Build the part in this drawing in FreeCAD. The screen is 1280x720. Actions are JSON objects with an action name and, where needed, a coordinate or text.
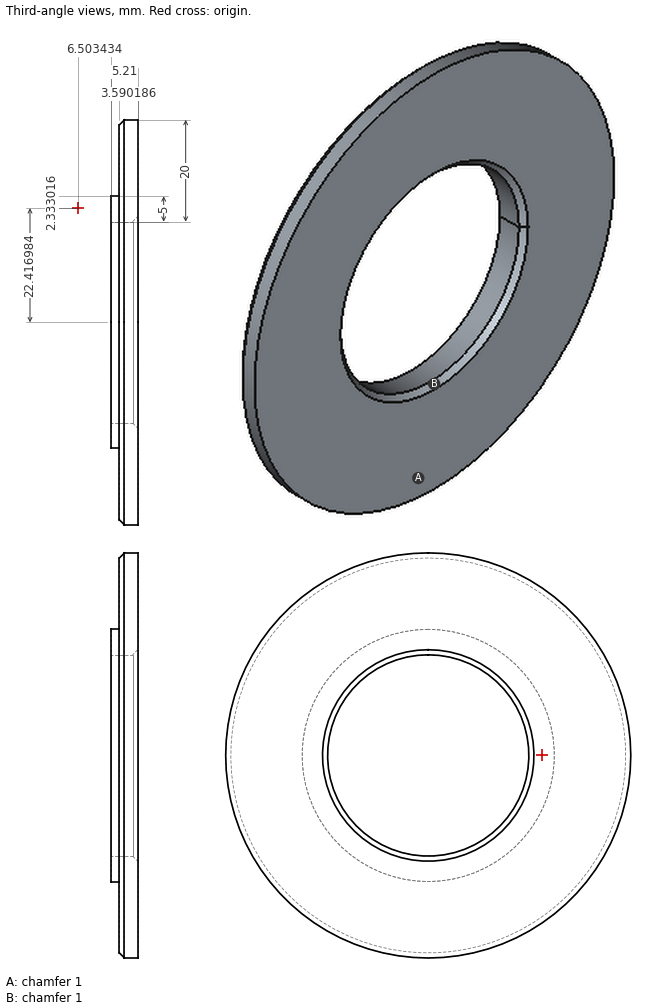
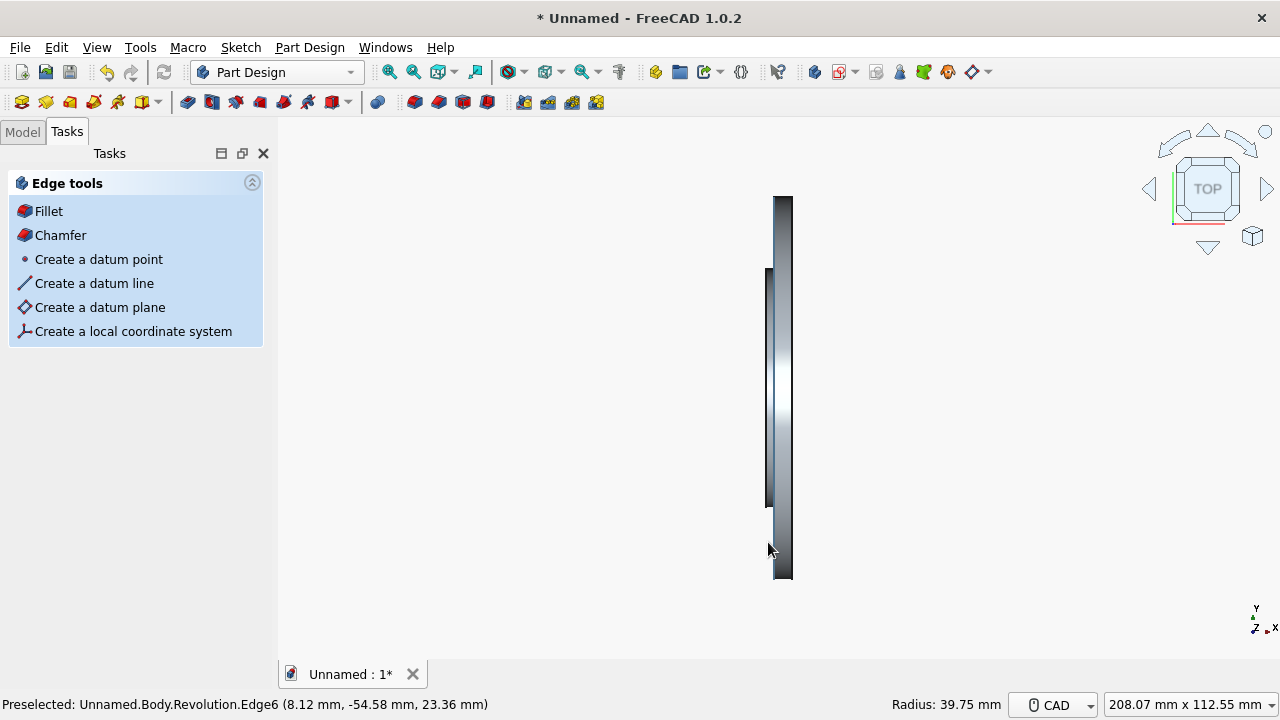
{"action": "left_click", "coordinate": [440, 102]}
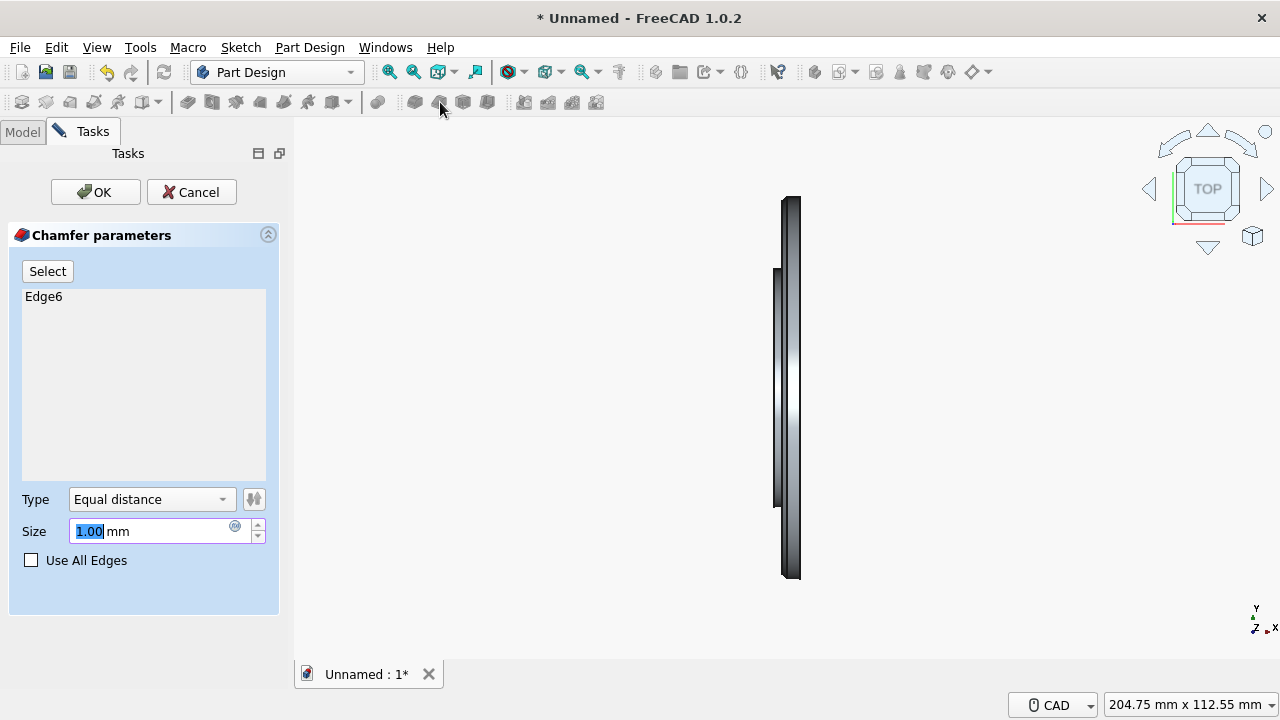
{"action": "type", "text": "1"}
{"action": "key", "text": "Tab"}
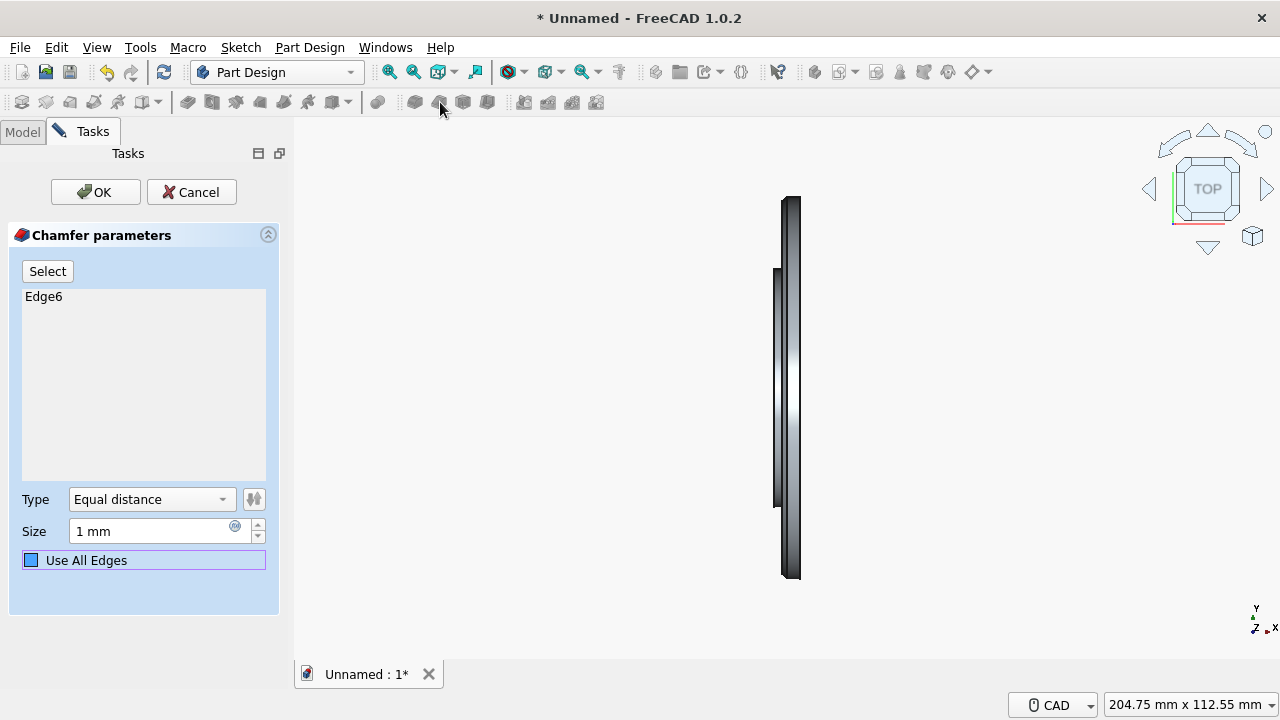
{"action": "left_click", "coordinate": [96, 192]}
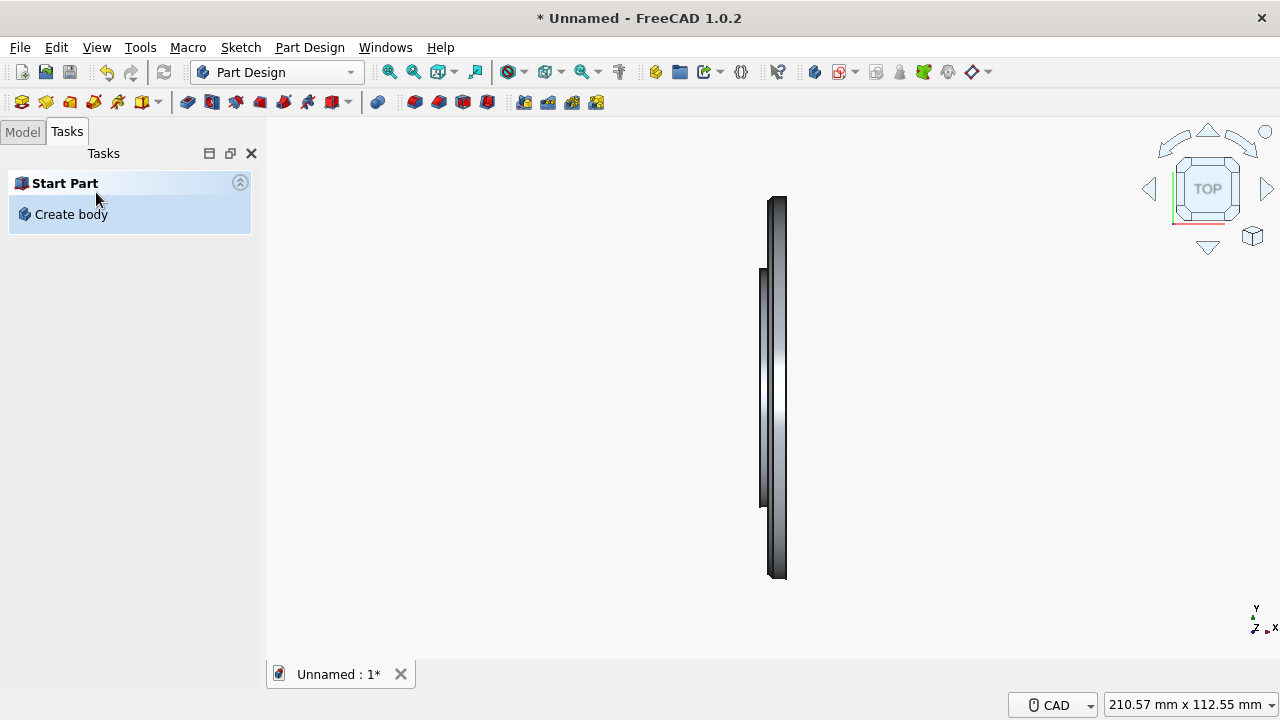
{"action": "key", "text": "0"}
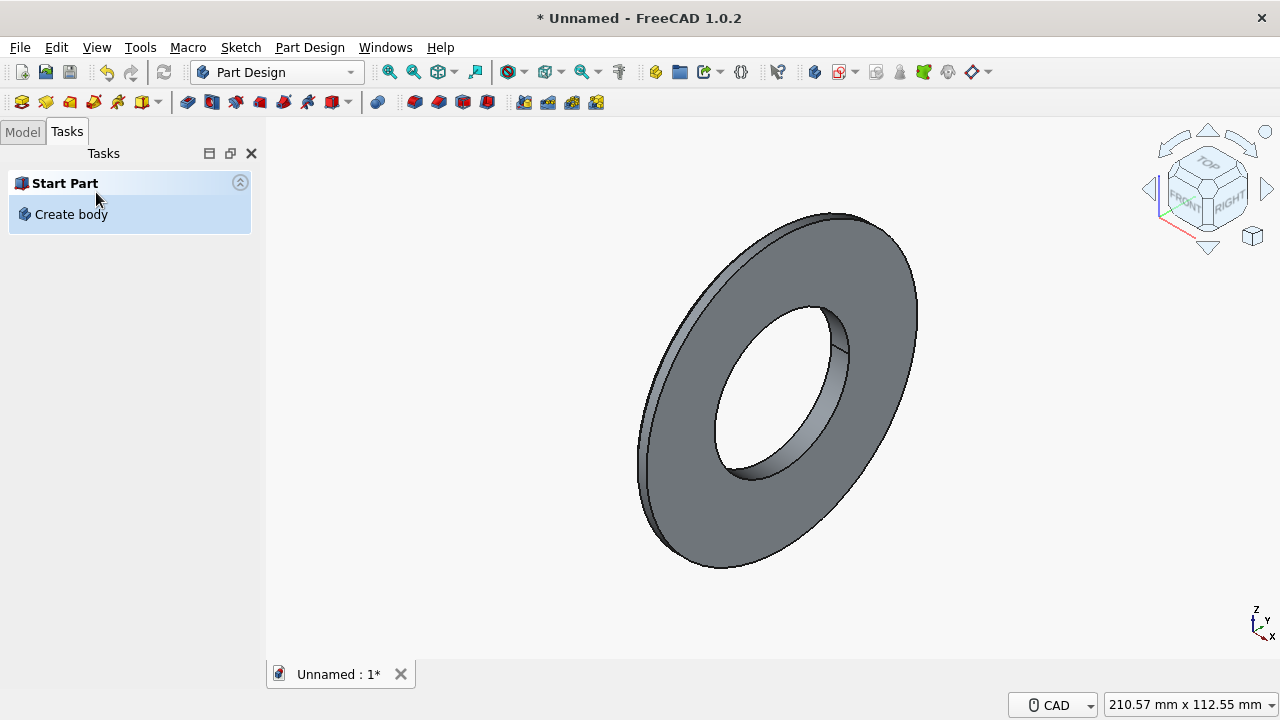
{"action": "left_click", "coordinate": [761, 478]}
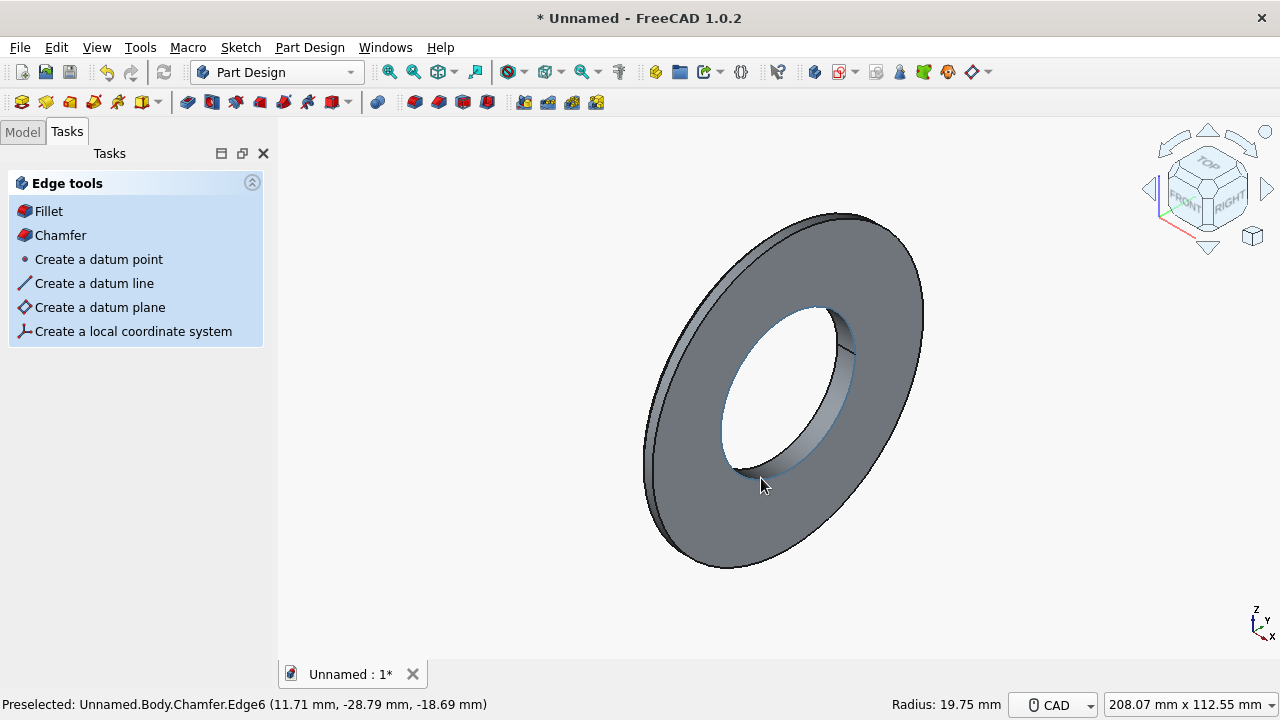
{"action": "left_click", "coordinate": [440, 102]}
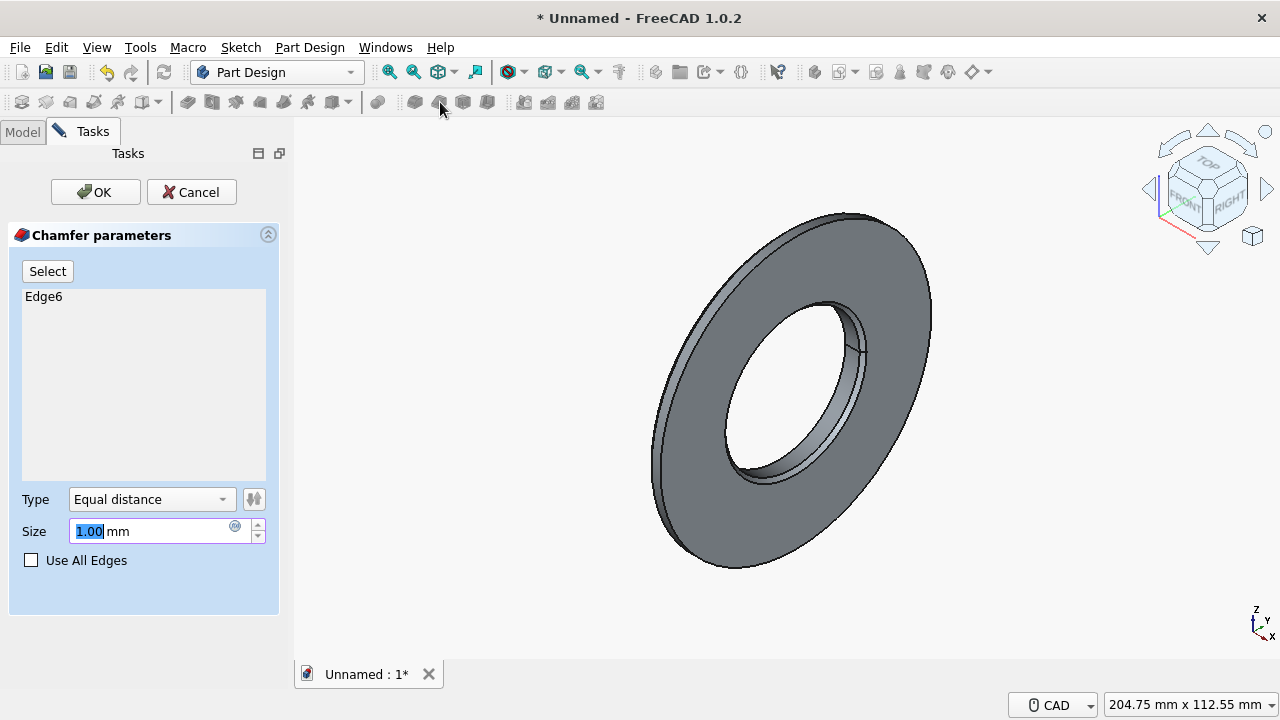
{"action": "type", "text": "1"}
{"action": "key", "text": "Tab"}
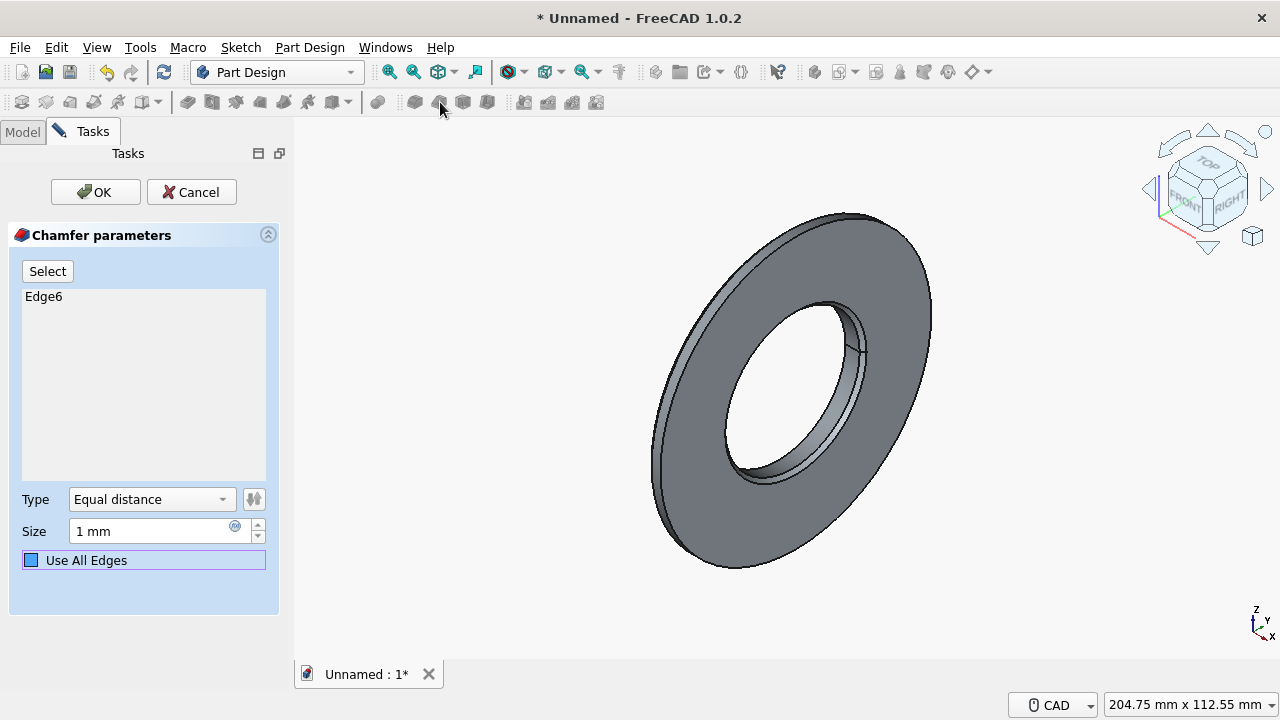
{"action": "left_click", "coordinate": [96, 192]}